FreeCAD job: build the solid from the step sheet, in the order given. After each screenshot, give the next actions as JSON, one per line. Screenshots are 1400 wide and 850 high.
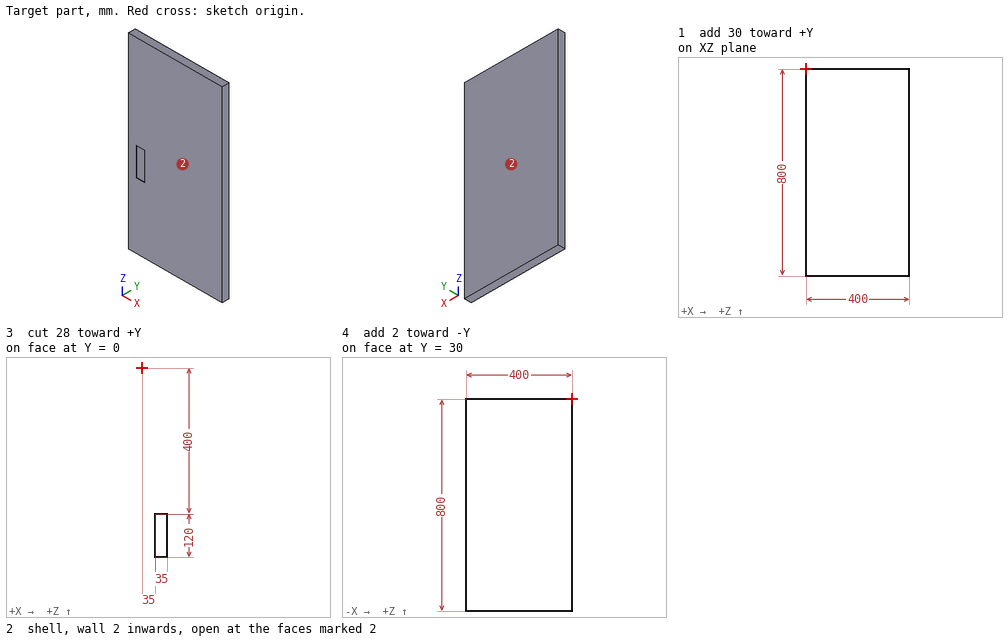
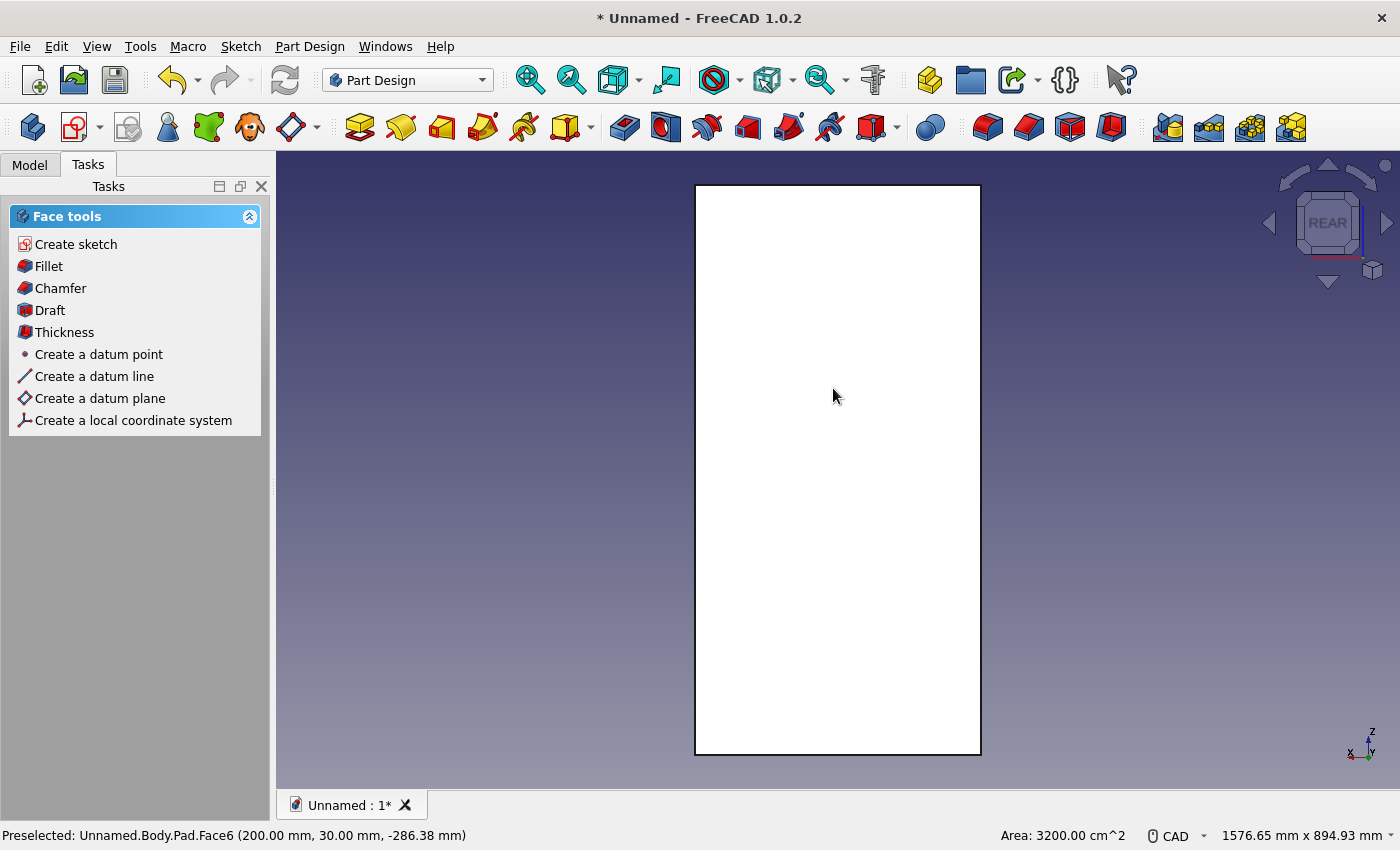
{"action": "left_click", "coordinate": [1111, 128]}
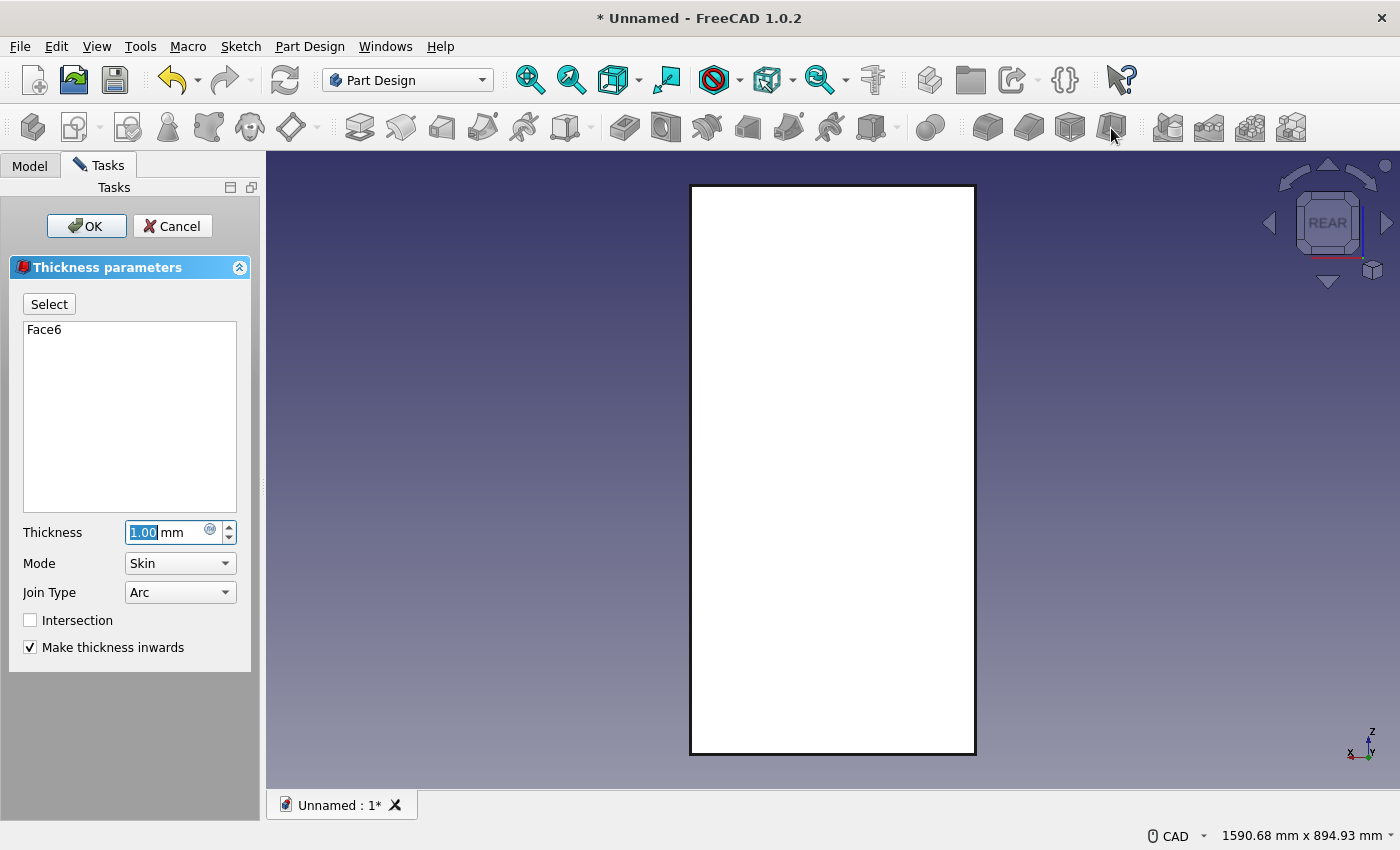
{"action": "type", "text": "2"}
{"action": "key", "text": "Tab"}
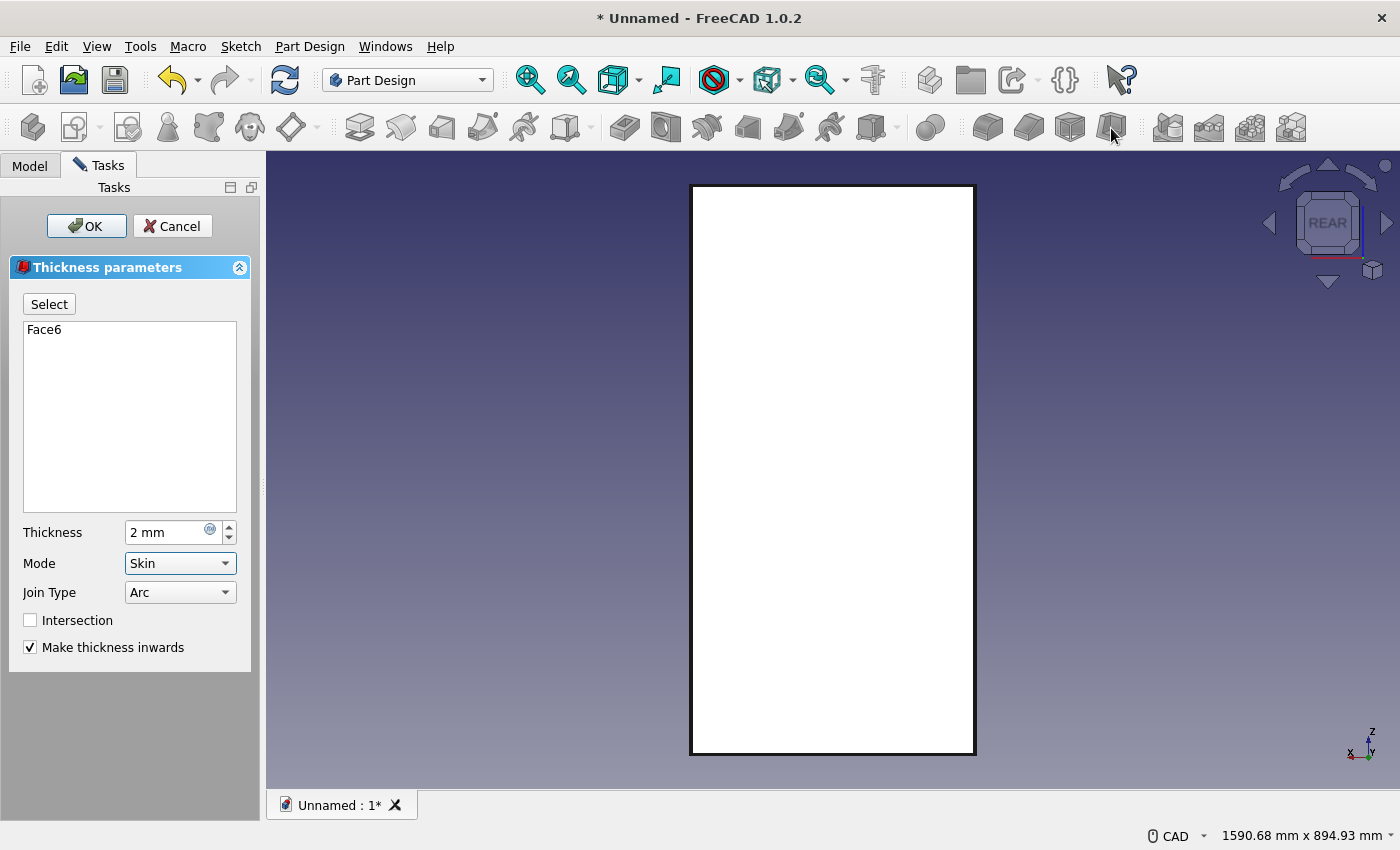
{"action": "left_click", "coordinate": [181, 592]}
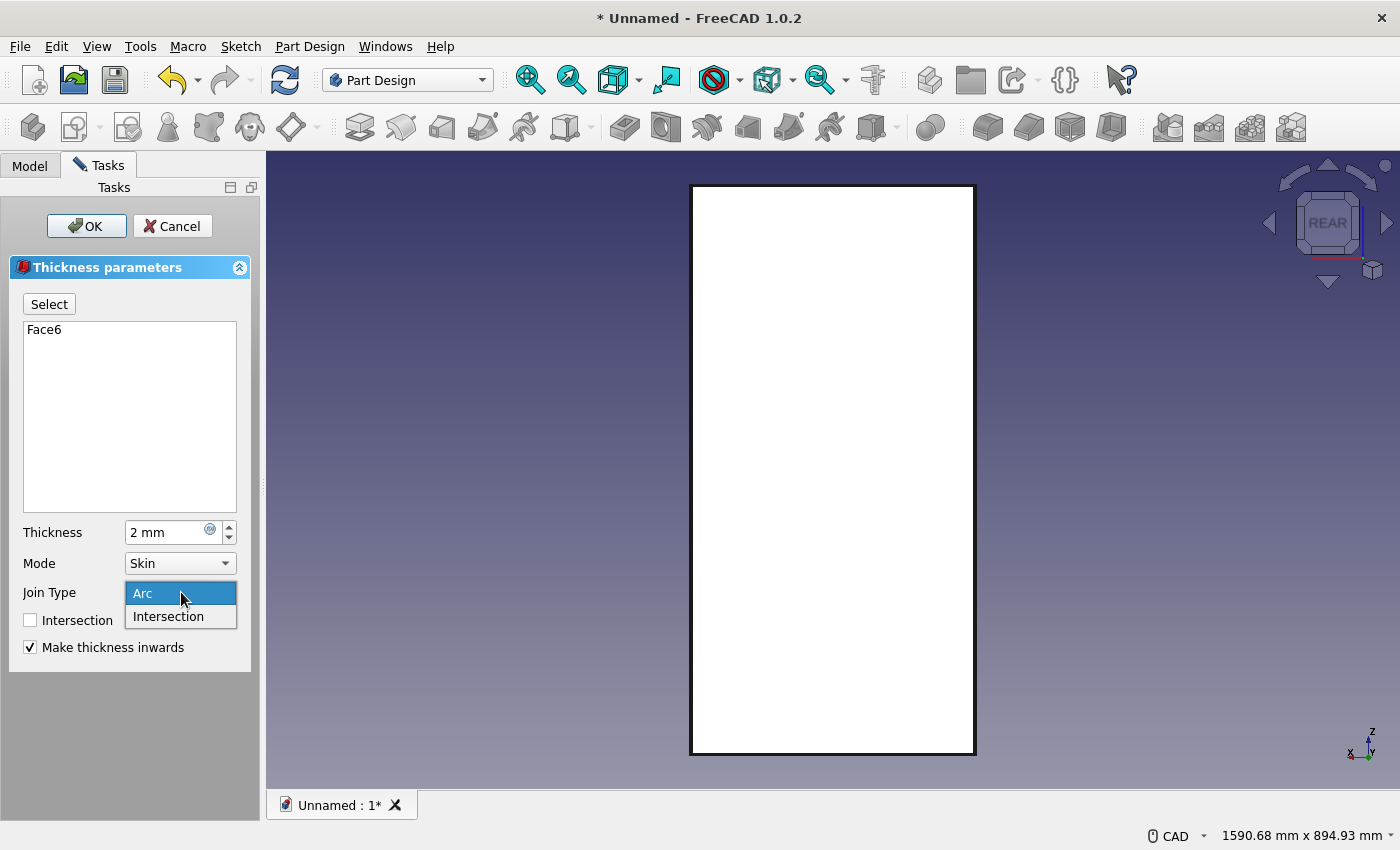
{"action": "left_click", "coordinate": [179, 616]}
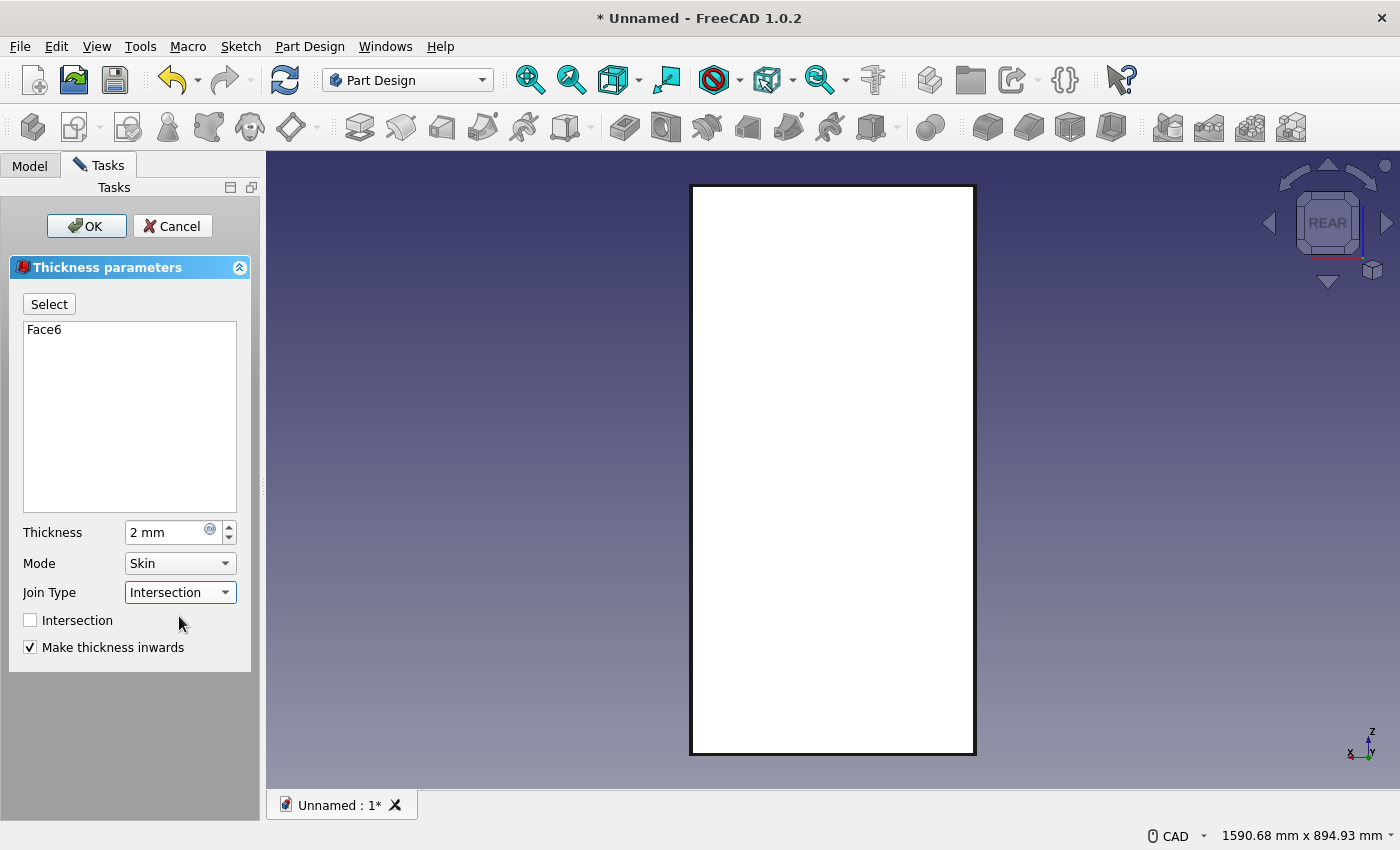
{"action": "left_click", "coordinate": [87, 226]}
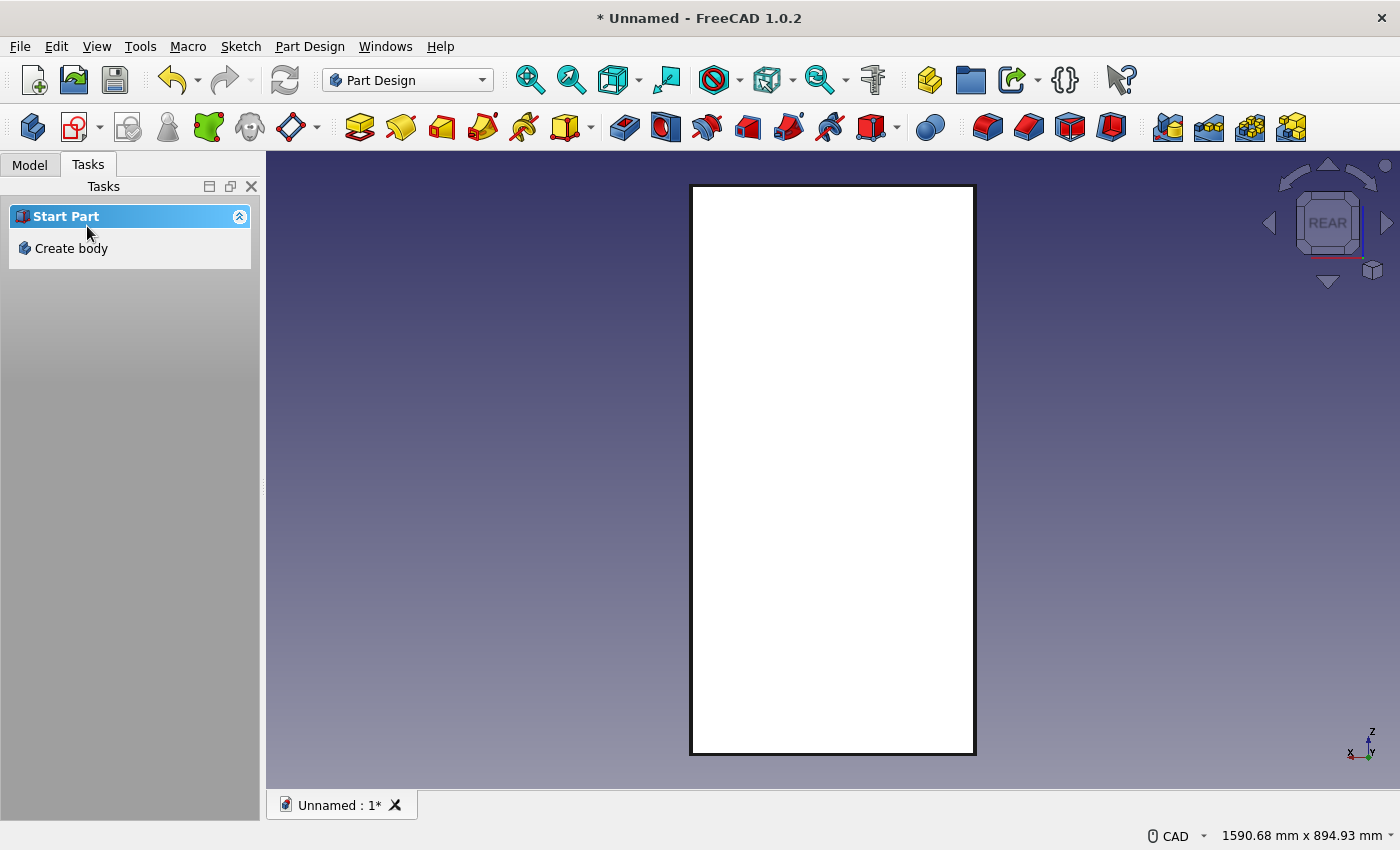
{"action": "key", "text": "0"}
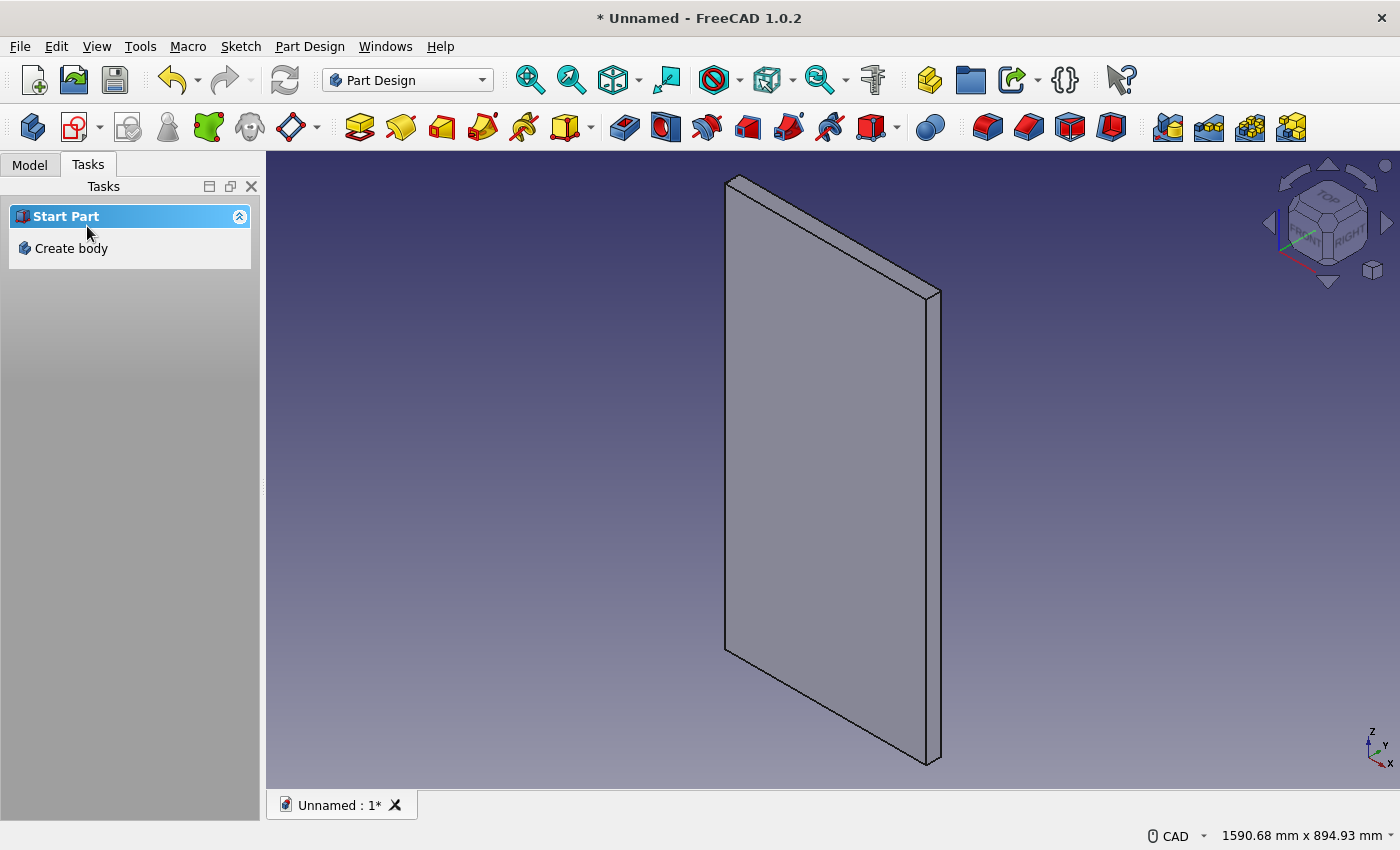
{"action": "left_click", "coordinate": [825, 407]}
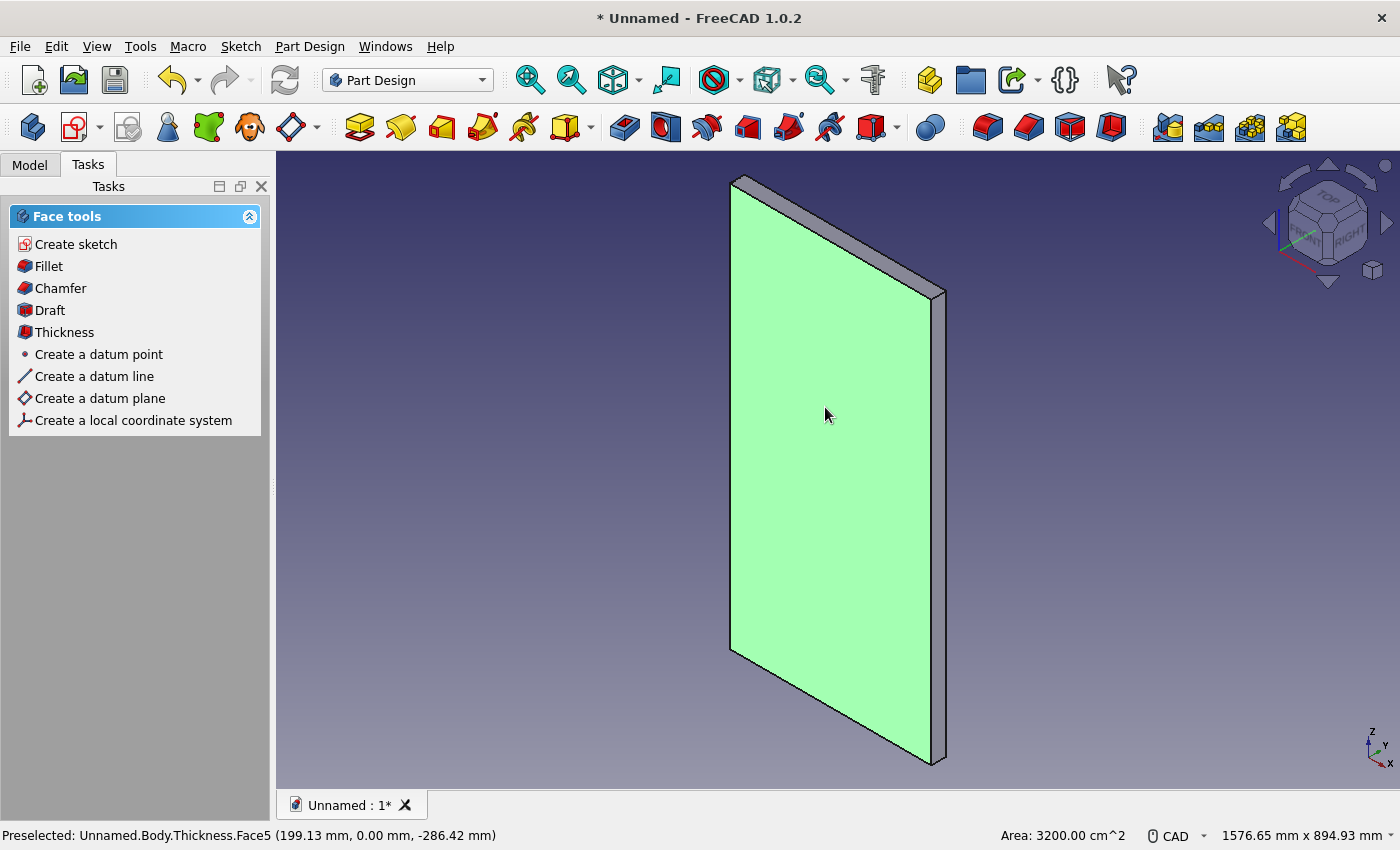
{"action": "left_click", "coordinate": [74, 128]}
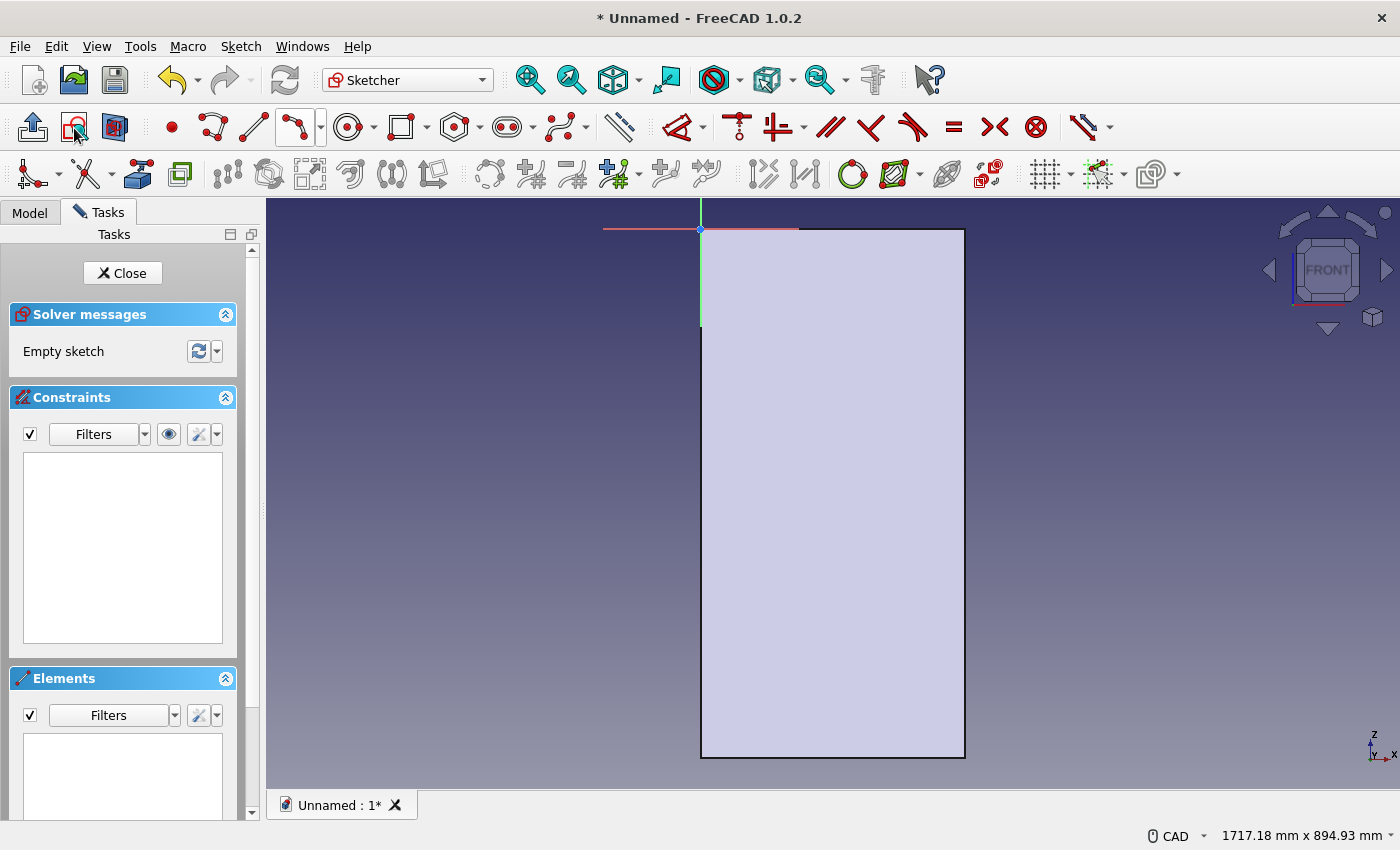
{"action": "scroll", "coordinate": [728, 543], "scroll_direction": "up", "scroll_amount": 8}